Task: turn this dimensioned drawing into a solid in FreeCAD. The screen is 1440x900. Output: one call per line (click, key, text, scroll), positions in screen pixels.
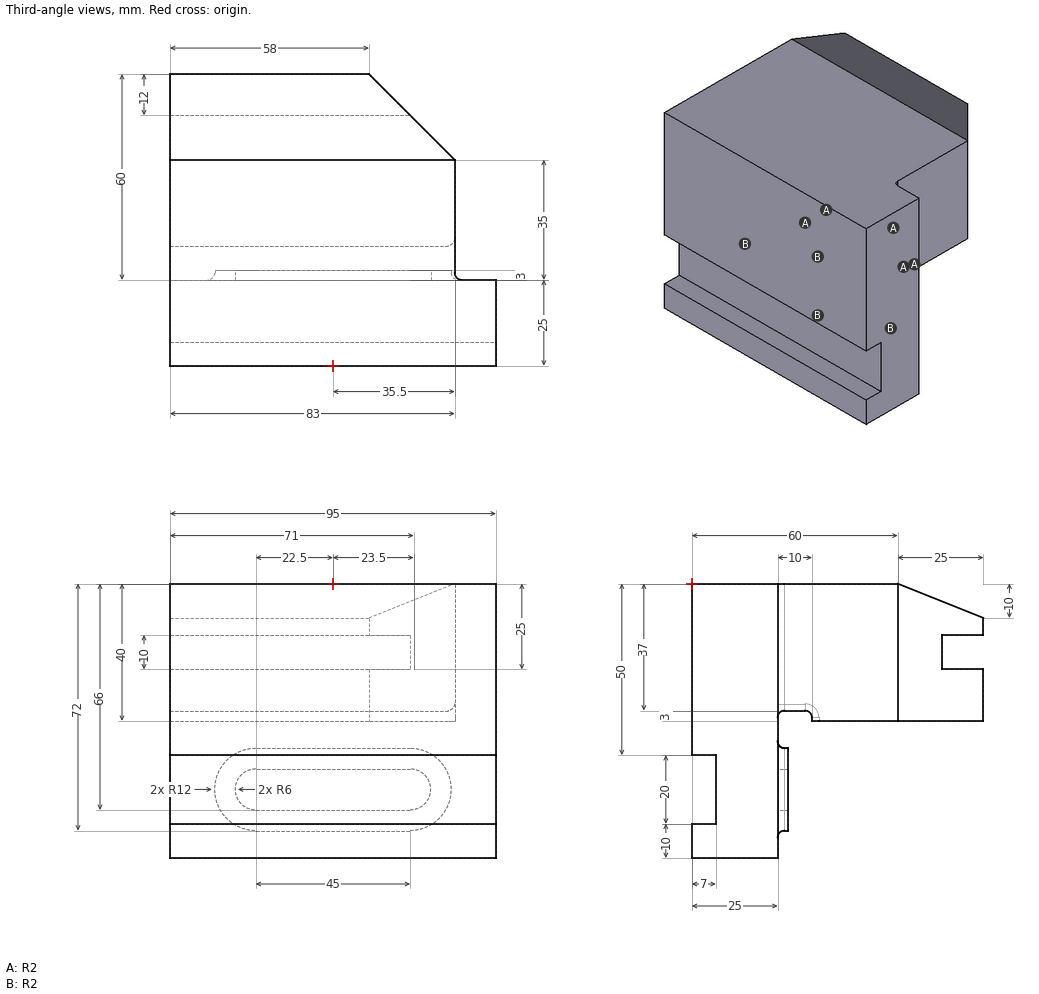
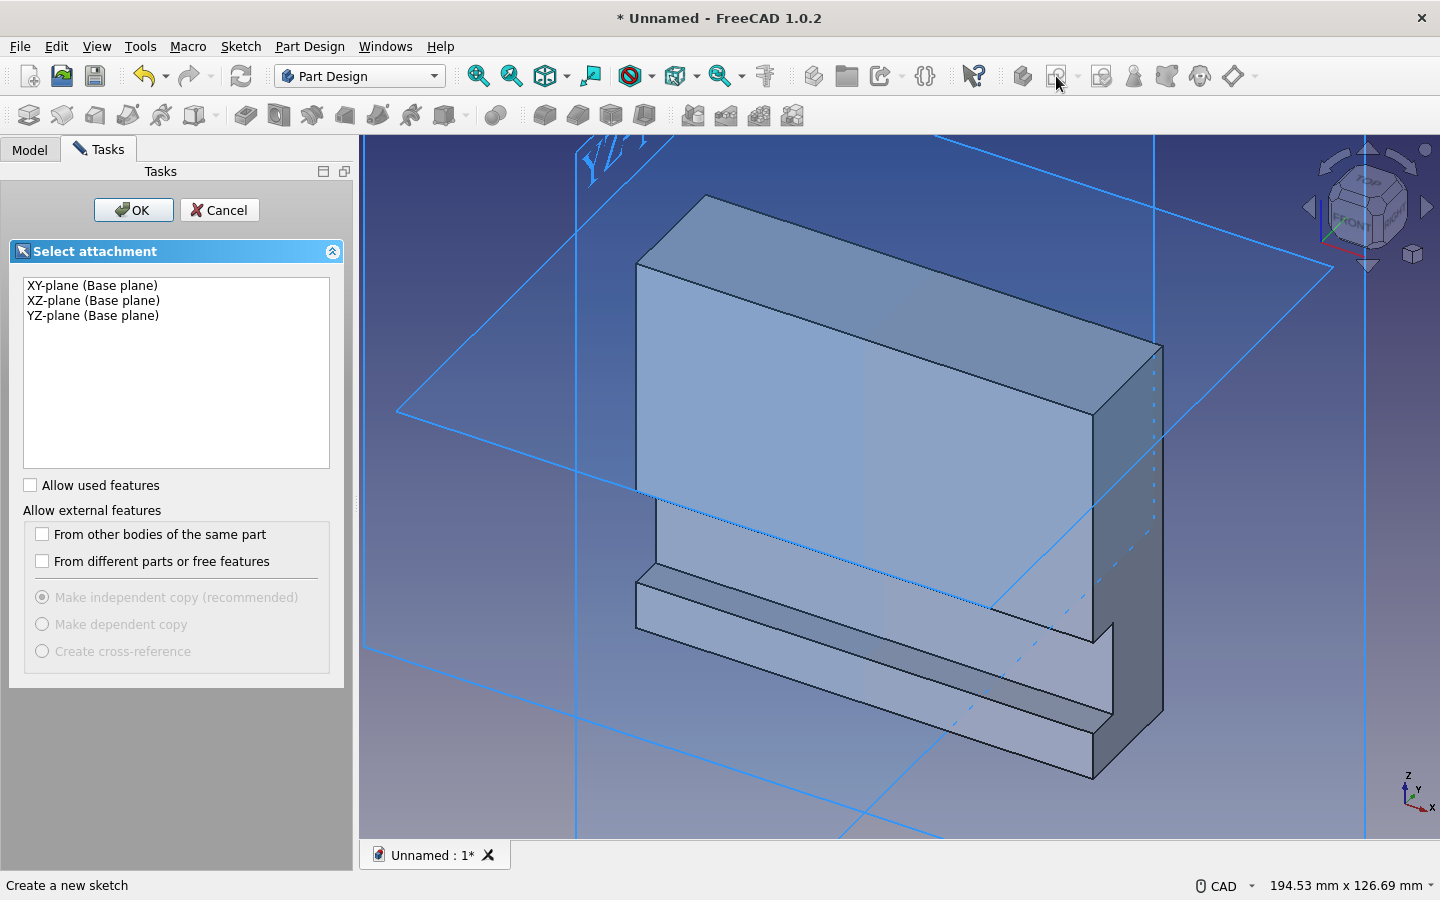
click(84, 286)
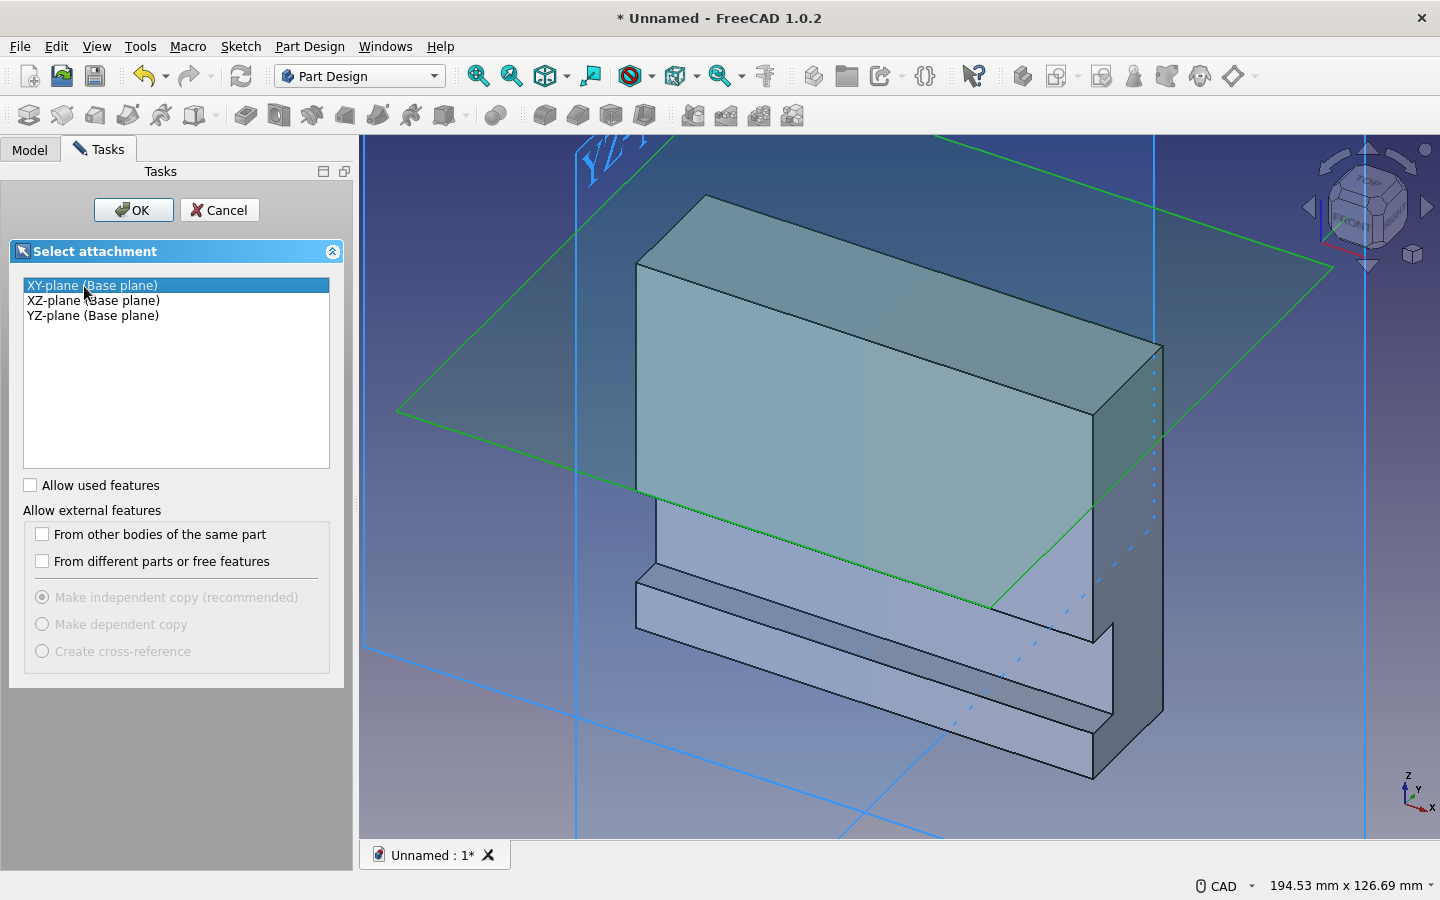
click(134, 210)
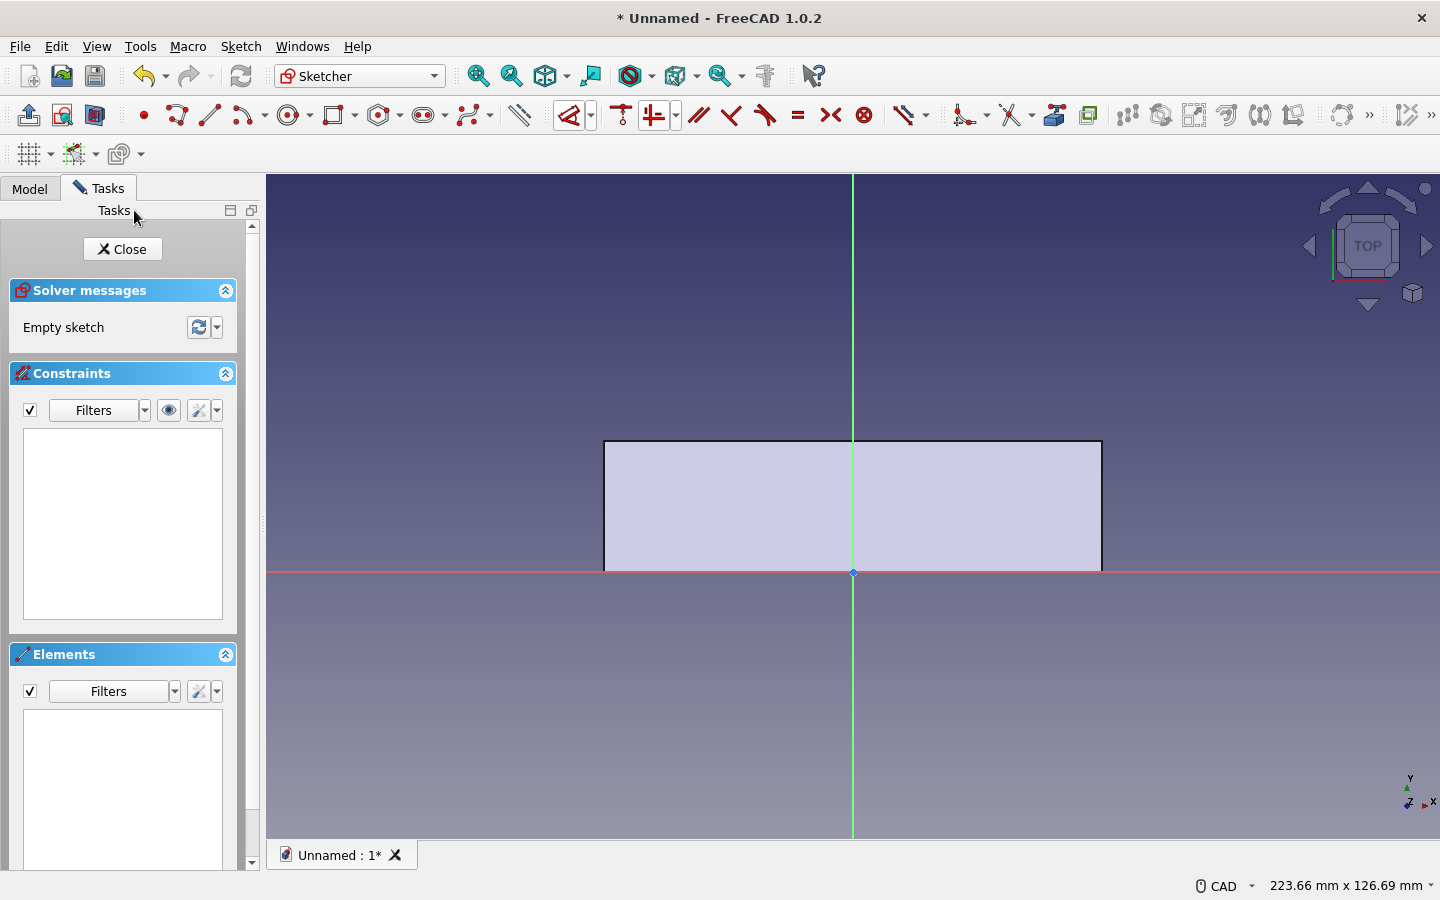
scroll(617, 811, down, 1)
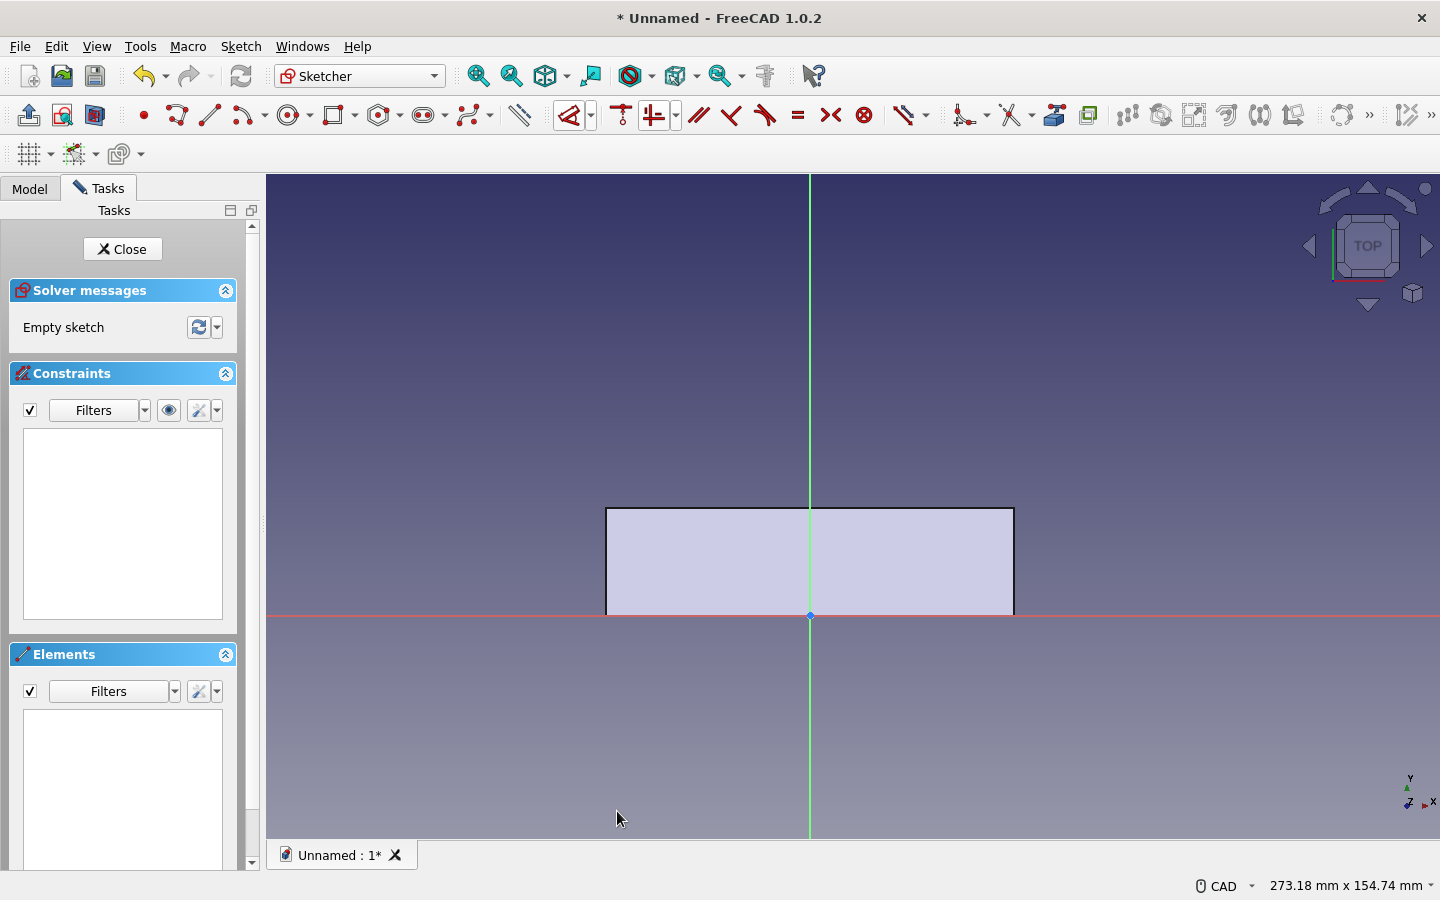
click(177, 116)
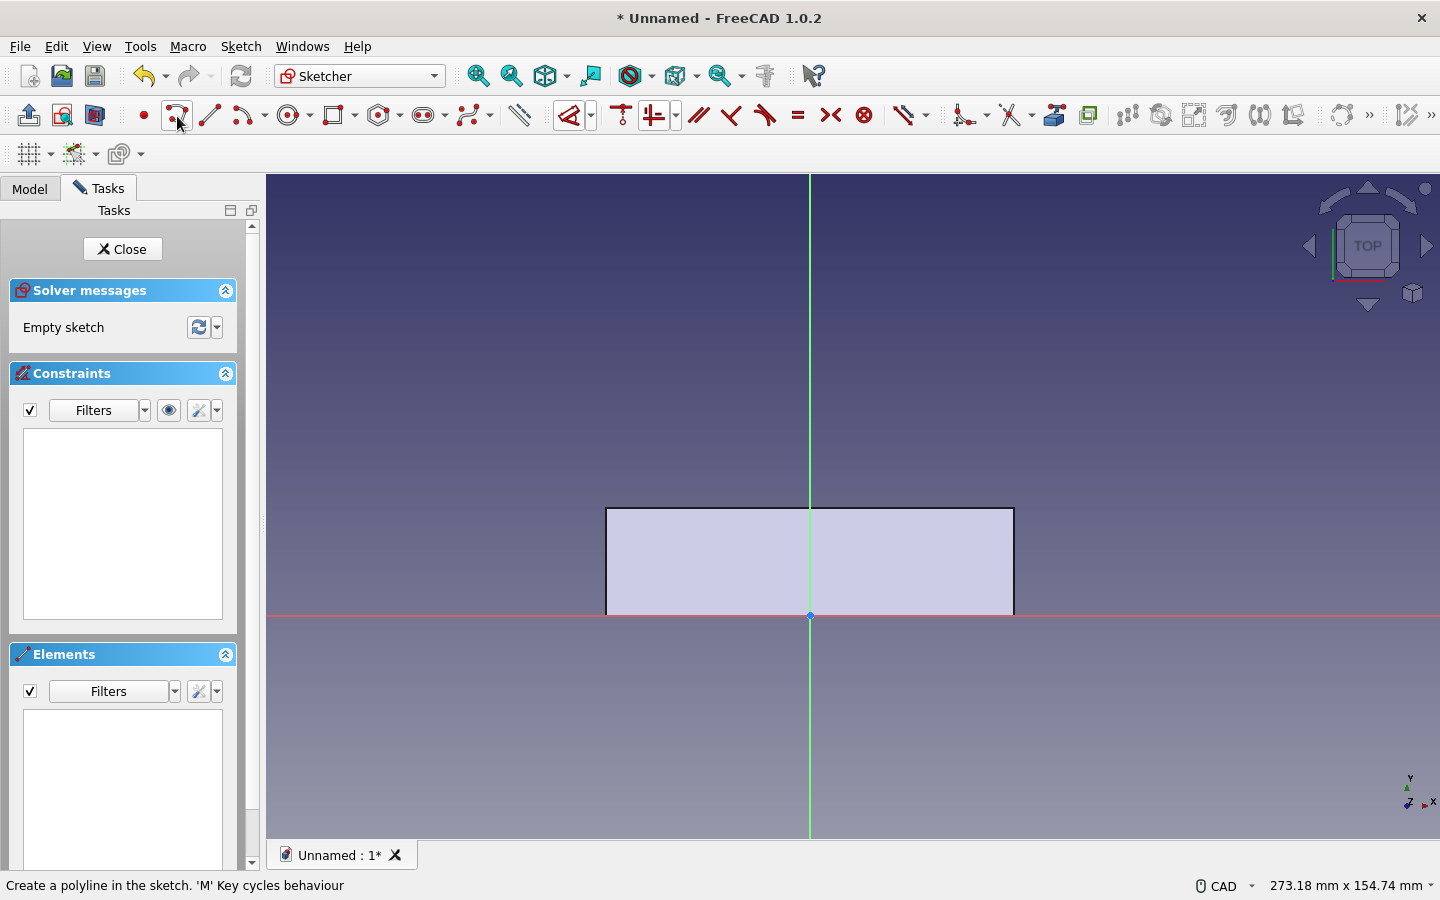
click(963, 508)
click(963, 358)
click(855, 250)
click(606, 250)
click(606, 508)
click(963, 509)
key(Escape)
key(Escape)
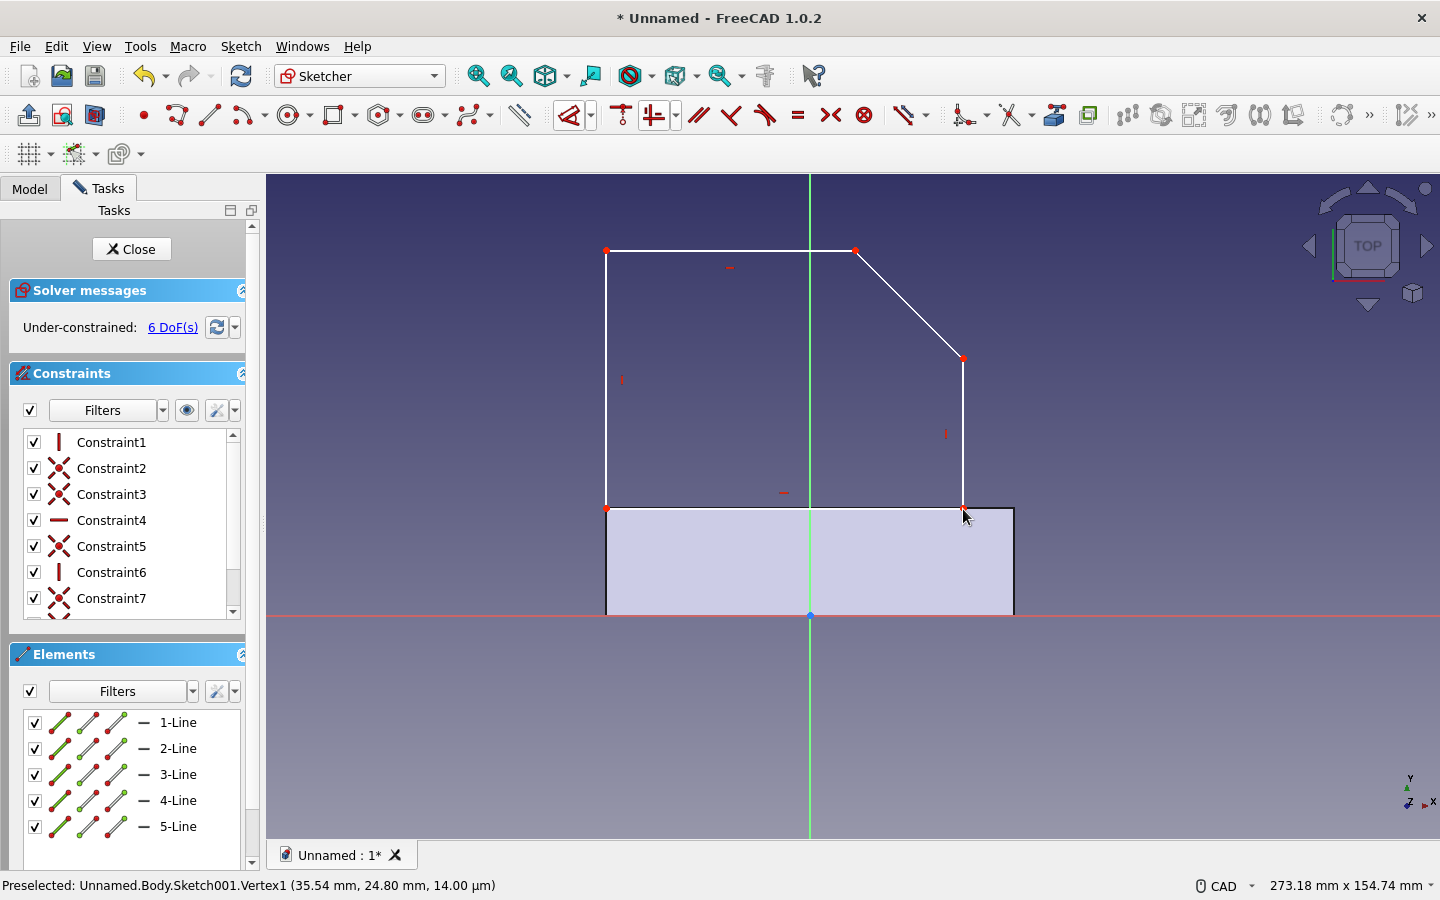
click(963, 464)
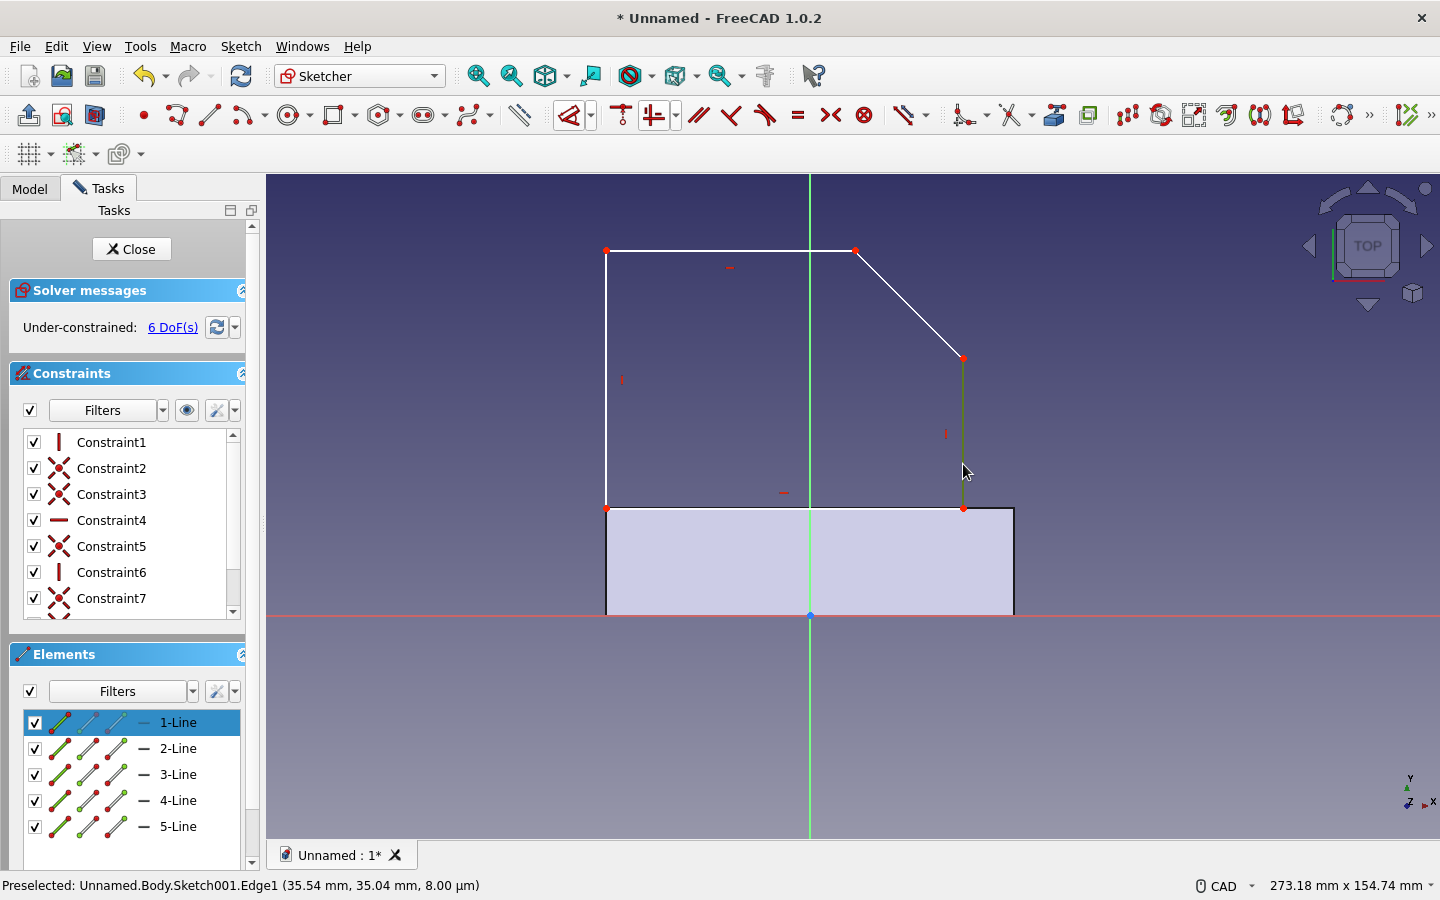
click(590, 116)